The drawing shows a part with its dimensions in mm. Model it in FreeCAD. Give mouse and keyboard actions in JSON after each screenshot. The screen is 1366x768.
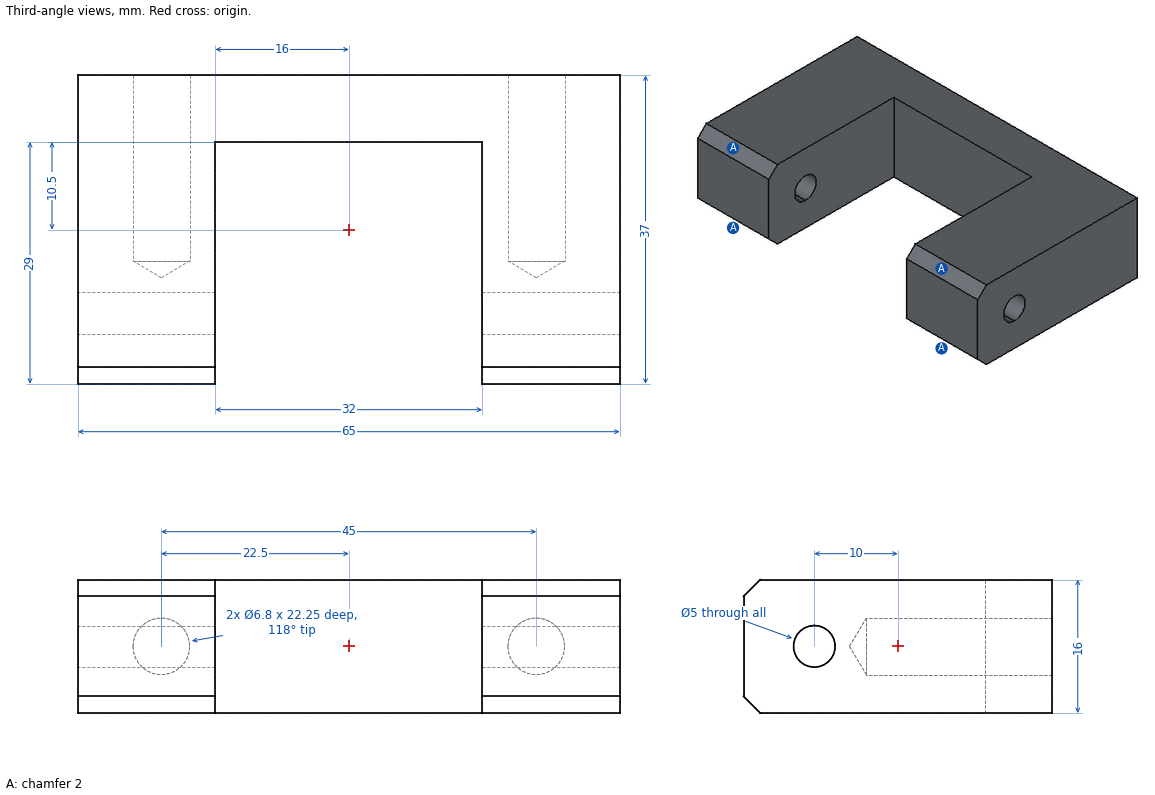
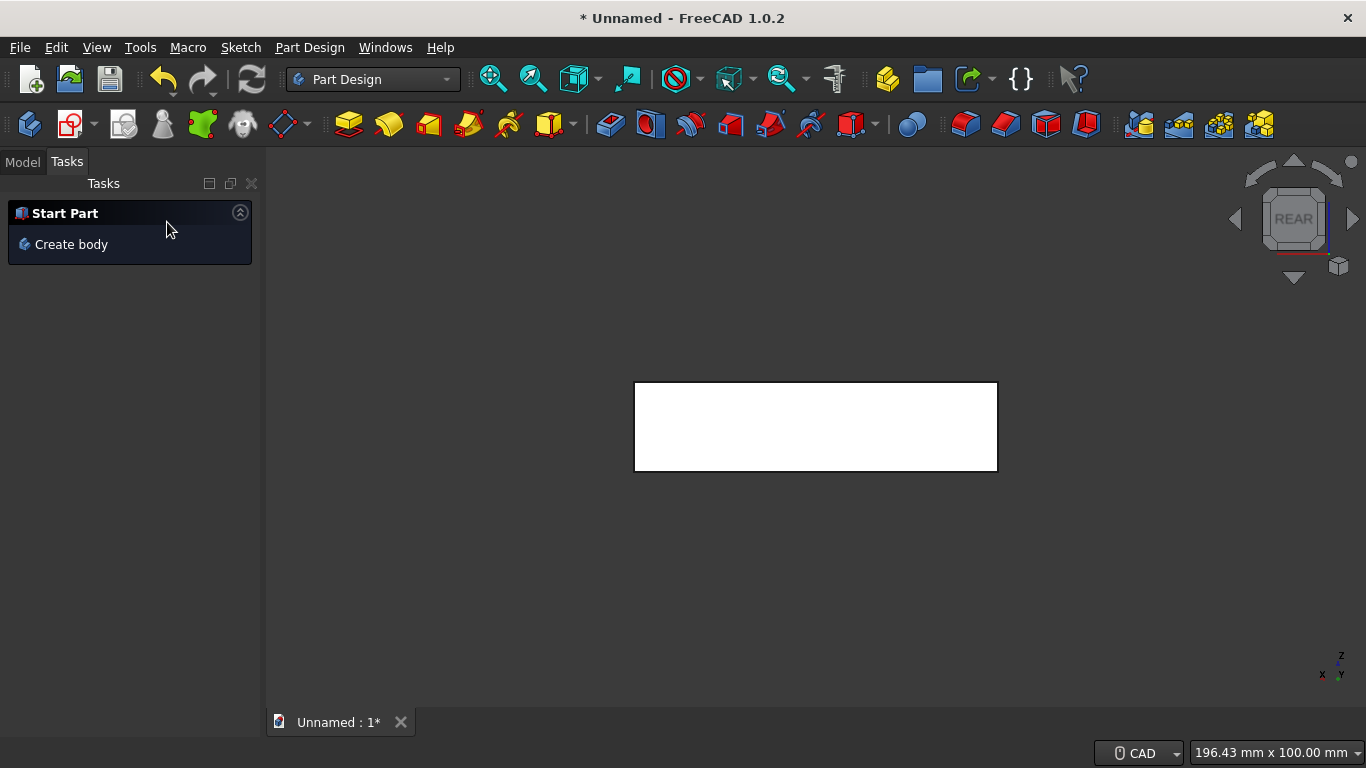
{"action": "left_click", "coordinate": [494, 80]}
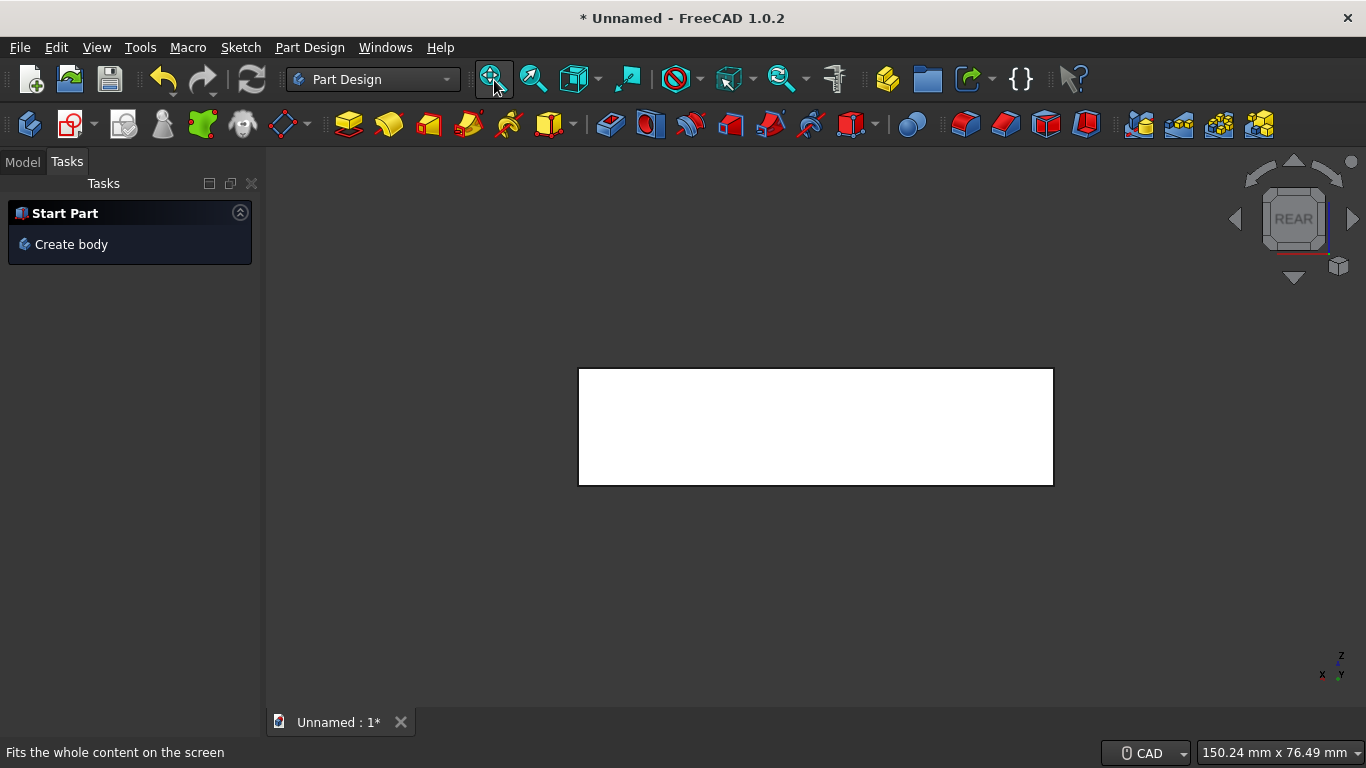
{"action": "left_click", "coordinate": [680, 426]}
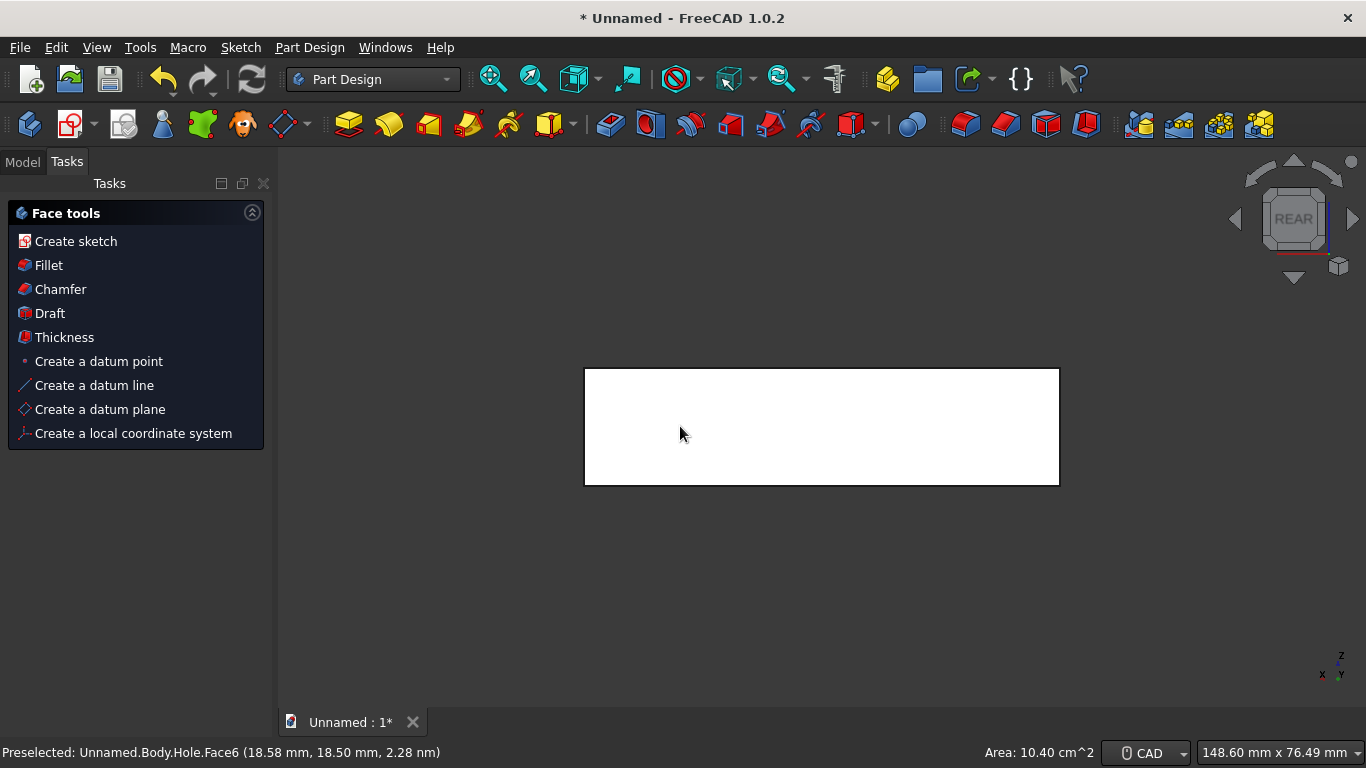
{"action": "left_click", "coordinate": [70, 124]}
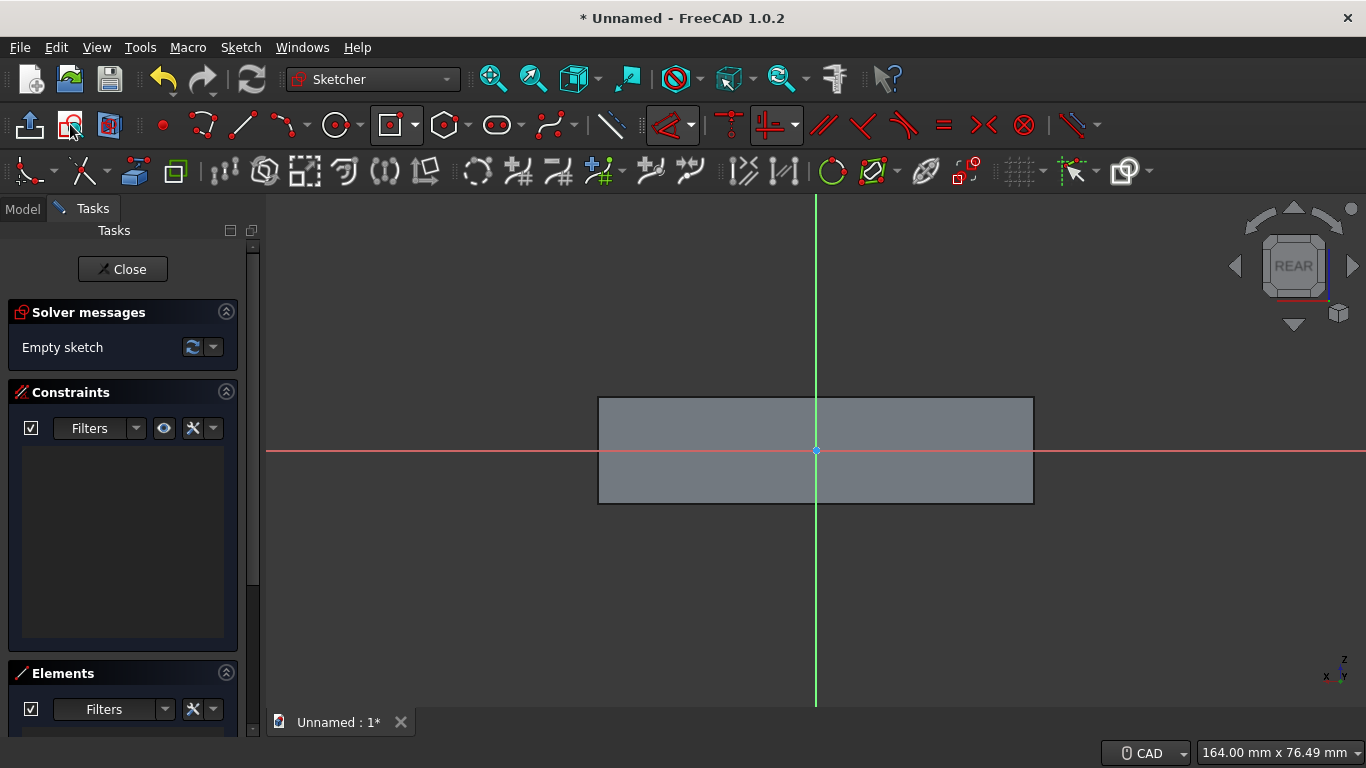
{"action": "scroll", "coordinate": [899, 450], "scroll_direction": "up", "scroll_amount": 3}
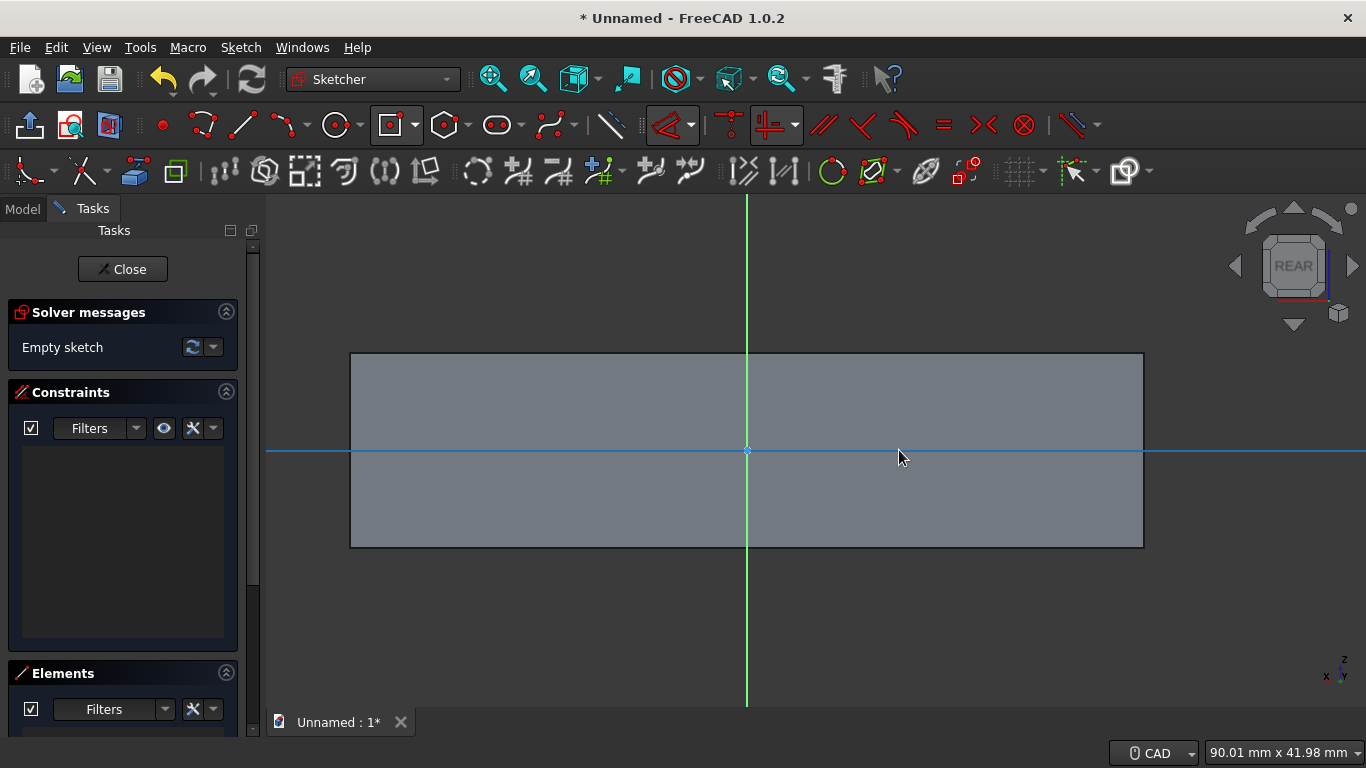
{"action": "left_click", "coordinate": [336, 126]}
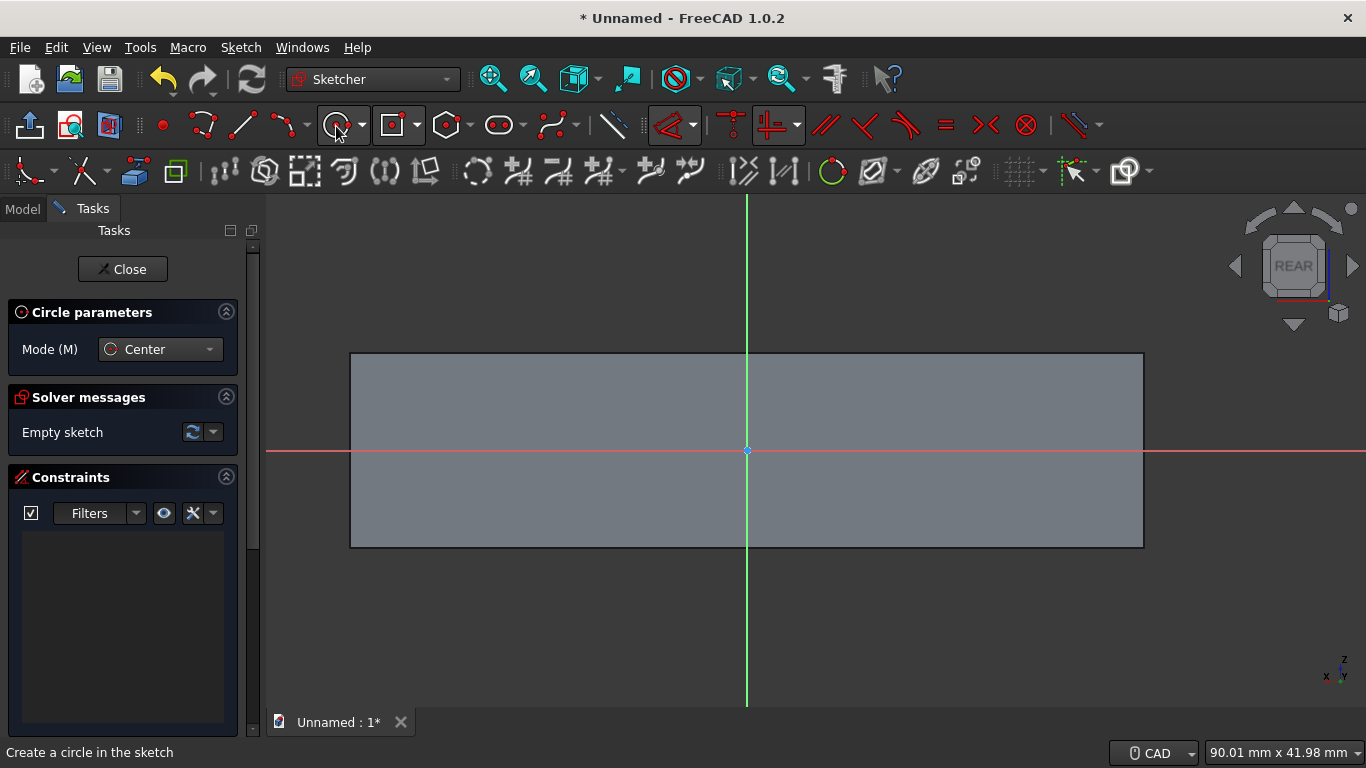
{"action": "left_click", "coordinate": [1022, 450]}
{"action": "left_click", "coordinate": [1052, 421]}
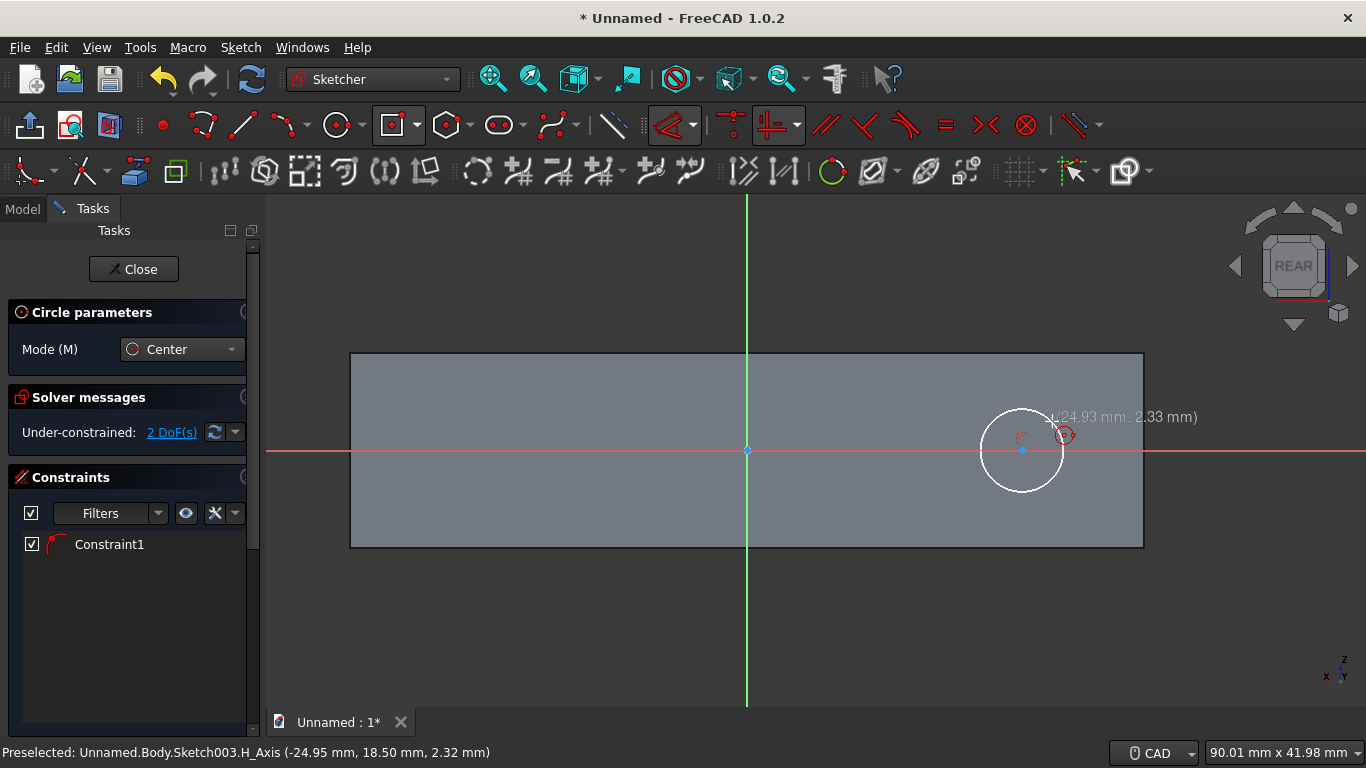
{"action": "left_click", "coordinate": [472, 450]}
{"action": "left_click", "coordinate": [502, 421]}
{"action": "key", "text": "Escape"}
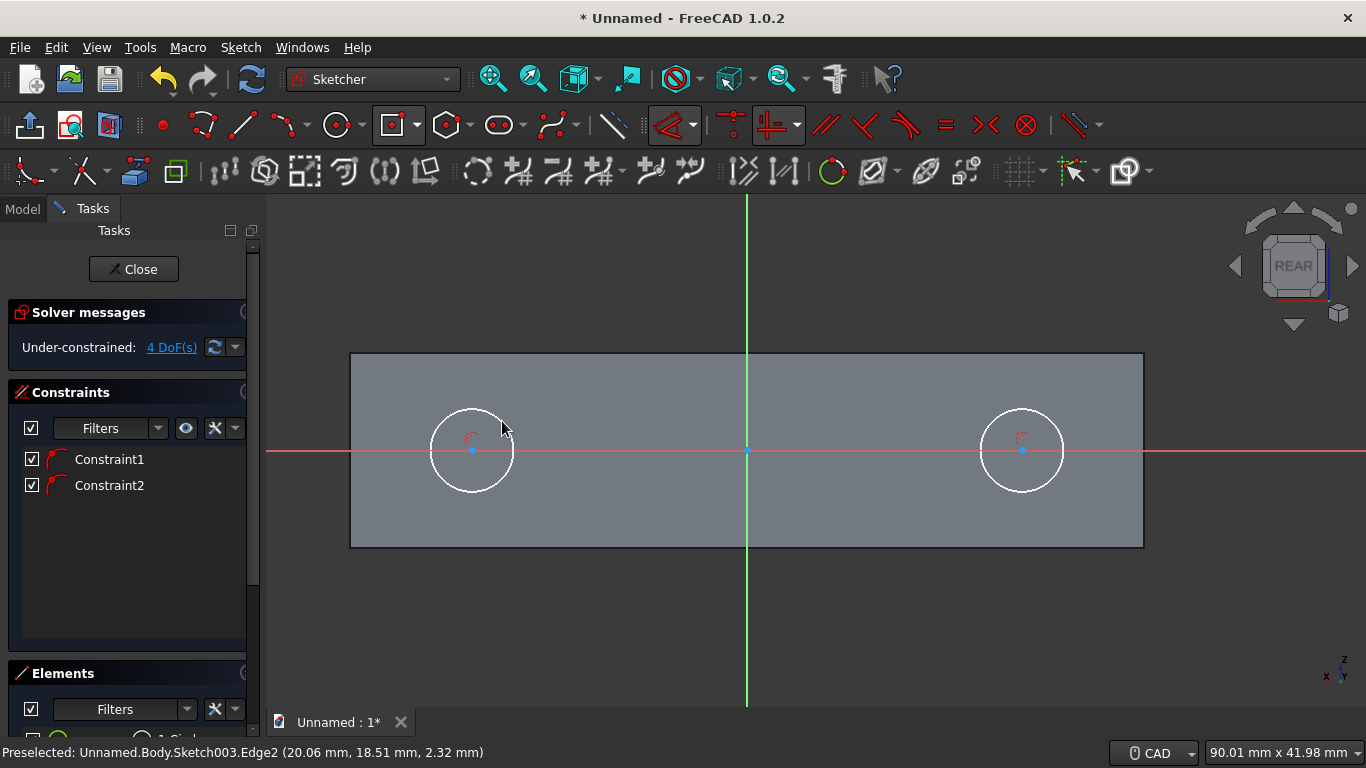
{"action": "left_click", "coordinate": [1051, 421]}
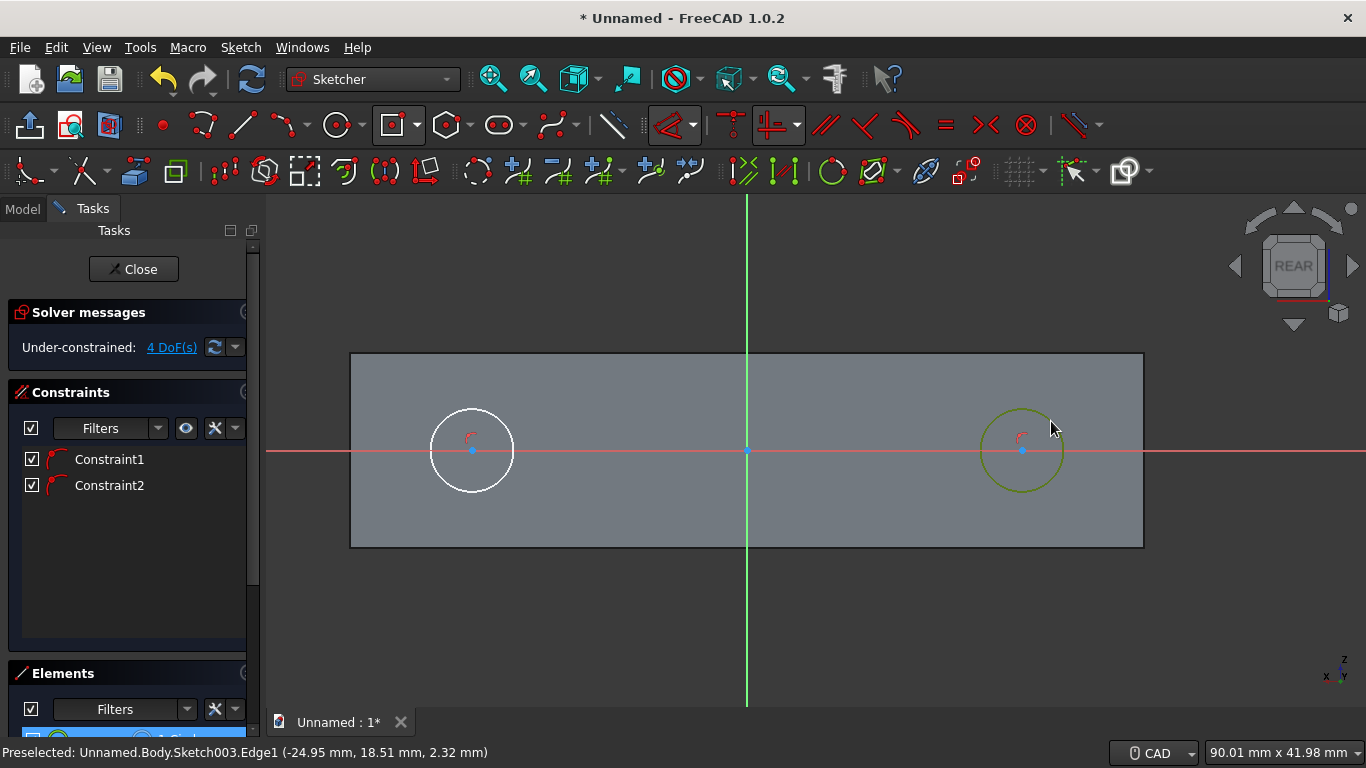
{"action": "left_click", "coordinate": [501, 421]}